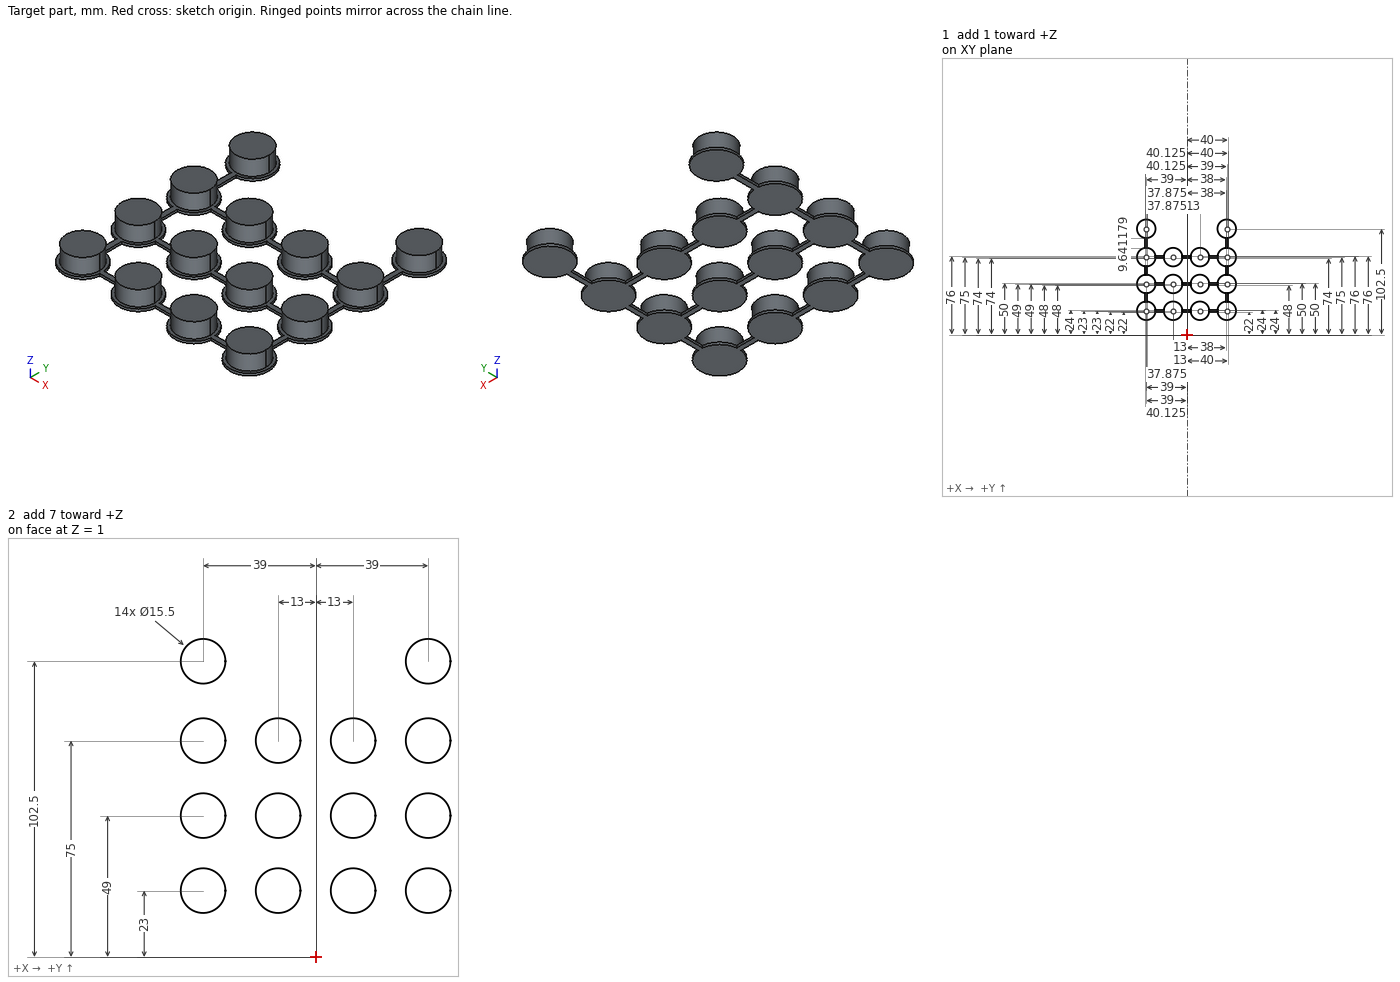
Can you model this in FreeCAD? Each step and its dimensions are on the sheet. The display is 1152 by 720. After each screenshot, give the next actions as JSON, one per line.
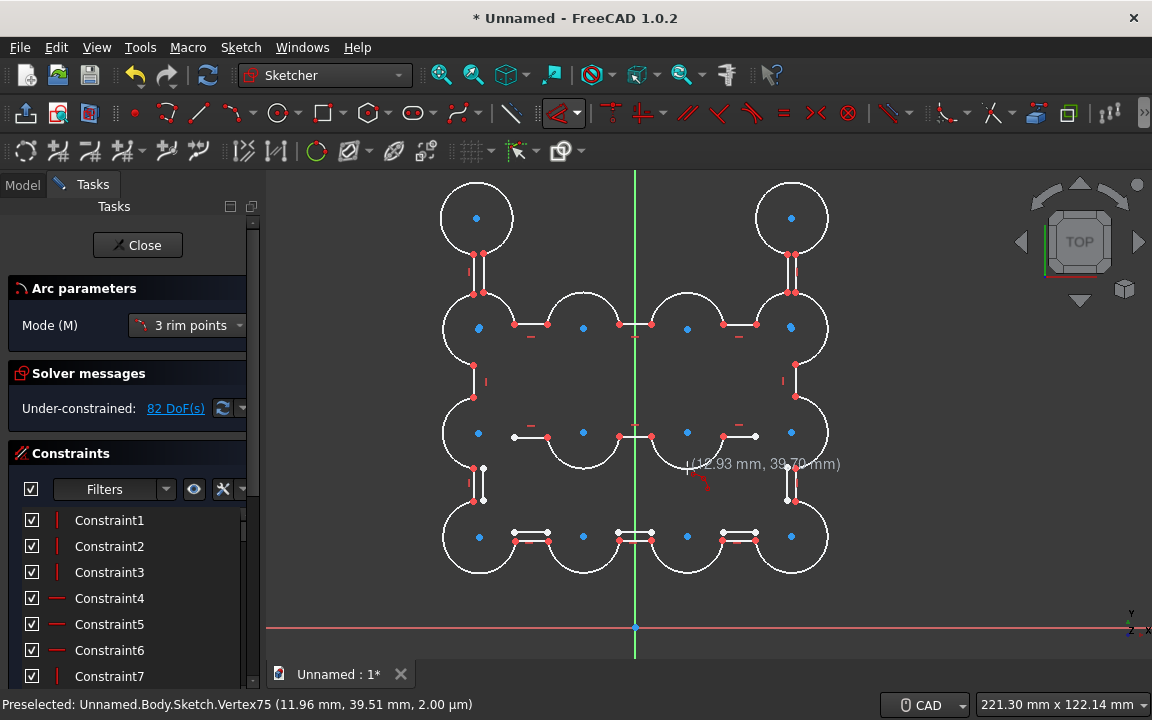
{"action": "left_click", "coordinate": [755, 437]}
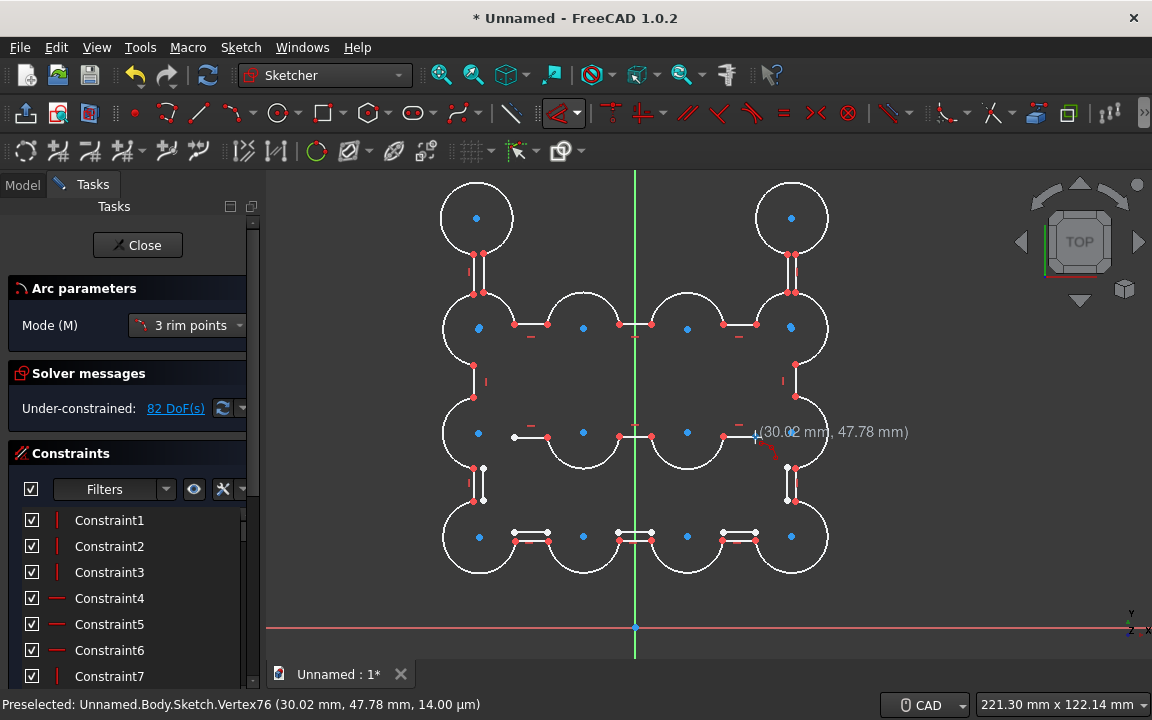
{"action": "scroll", "coordinate": [787, 468], "scroll_direction": "up", "scroll_amount": 4}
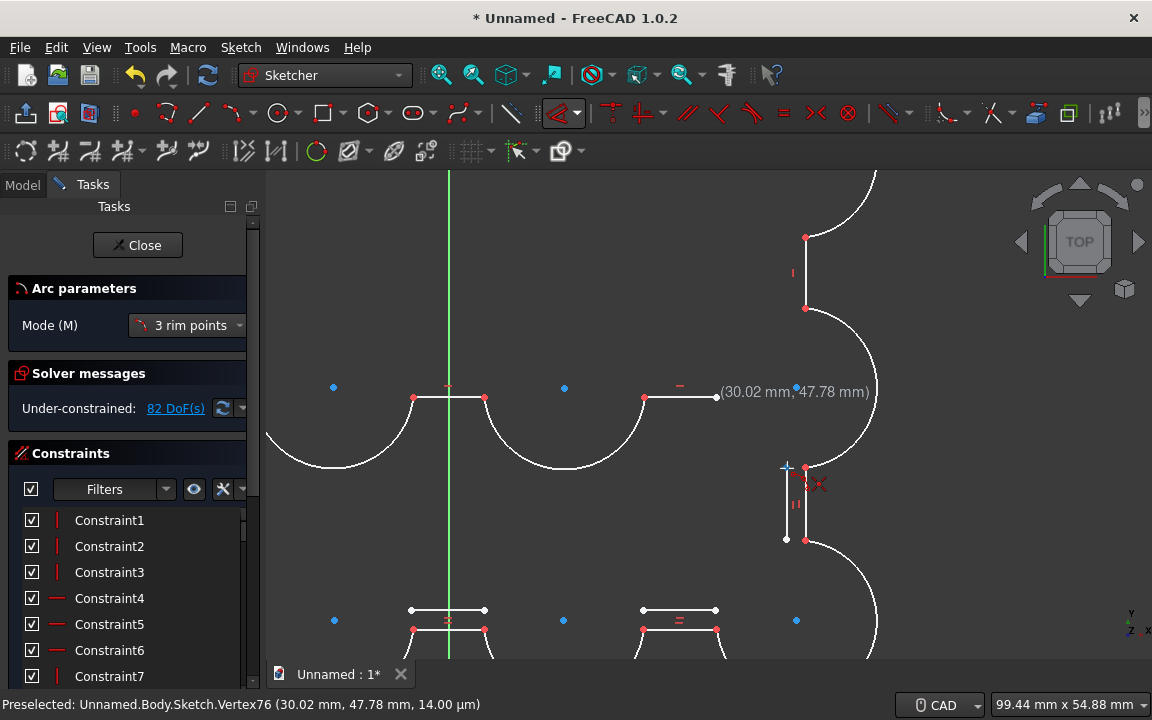
{"action": "left_click", "coordinate": [787, 467]}
{"action": "left_click", "coordinate": [739, 443]}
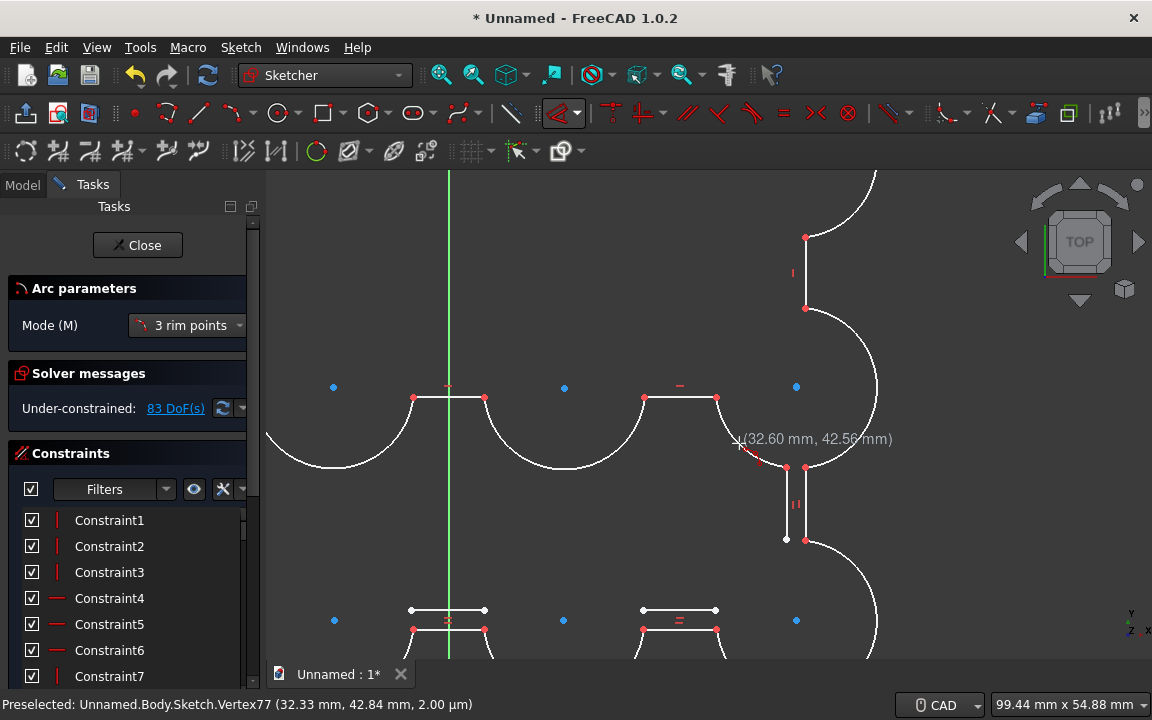
{"action": "left_click", "coordinate": [787, 539]}
{"action": "left_click", "coordinate": [716, 610]}
{"action": "left_click", "coordinate": [739, 562]}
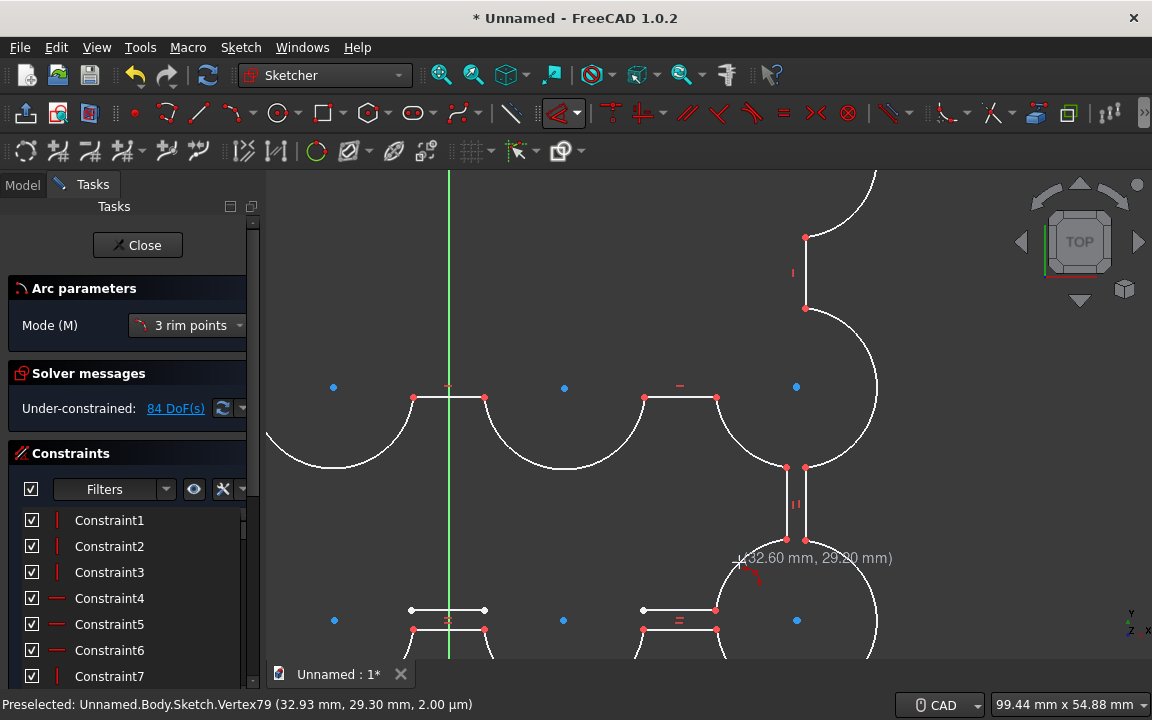
{"action": "left_click", "coordinate": [644, 610]}
{"action": "left_click", "coordinate": [485, 610]}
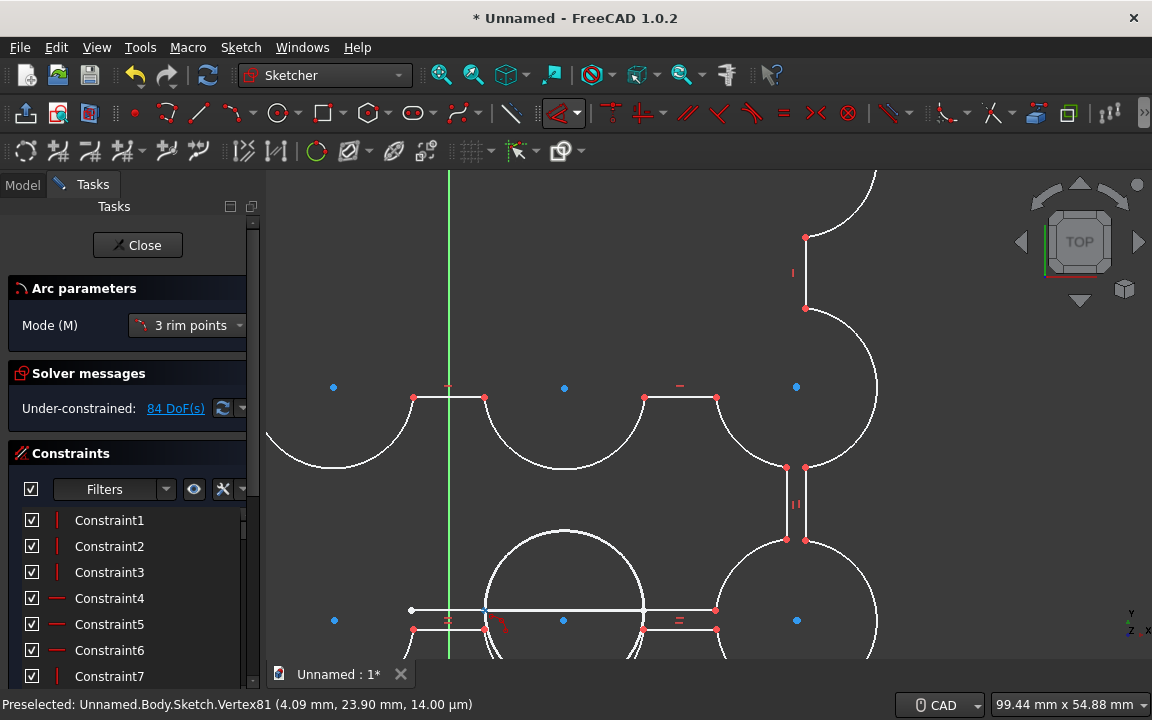
{"action": "scroll", "coordinate": [723, 452], "scroll_direction": "down", "scroll_amount": 6}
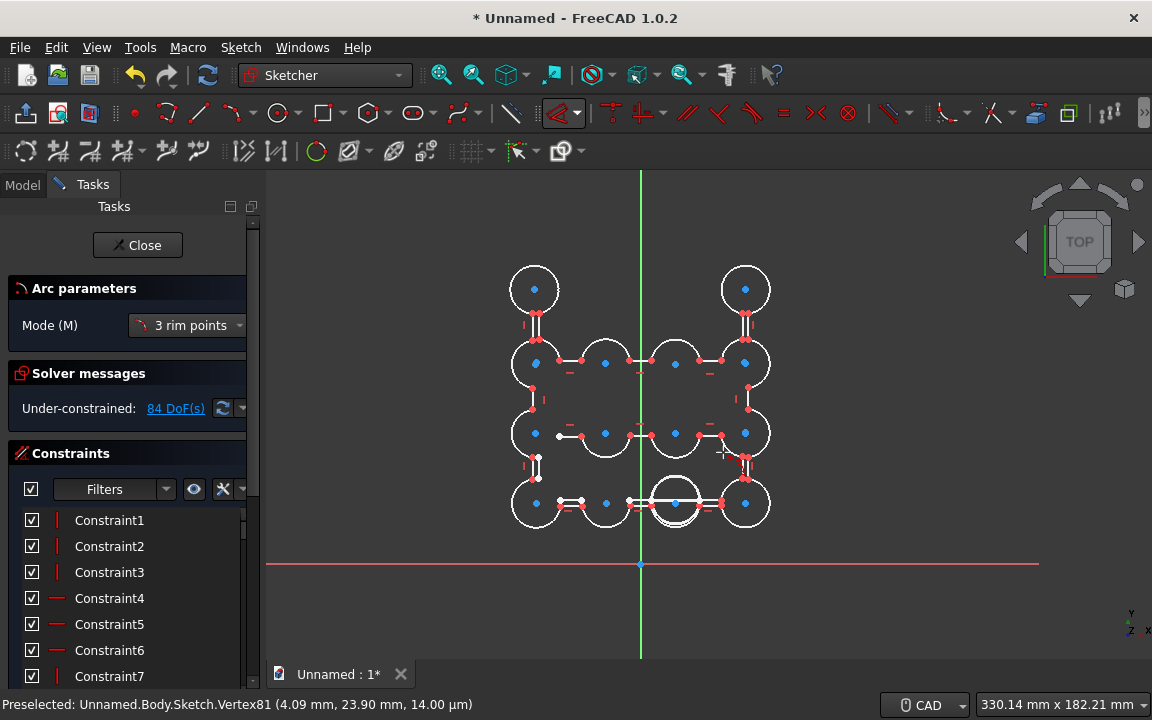
{"action": "left_click", "coordinate": [676, 478]}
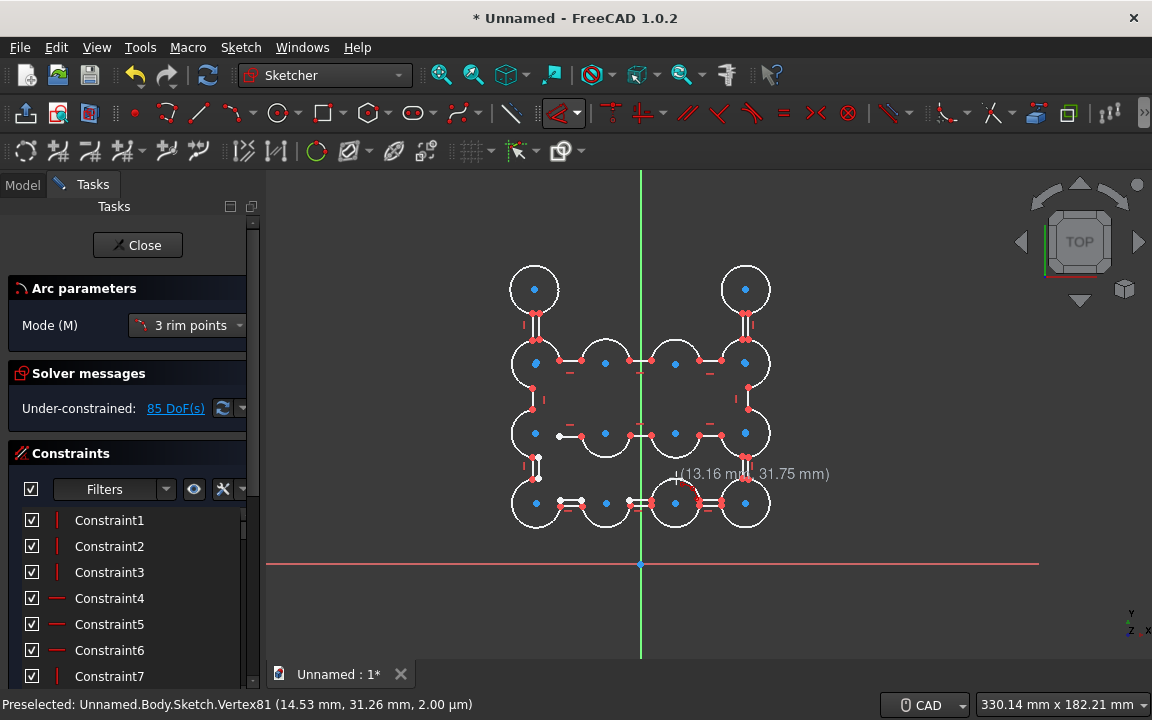
{"action": "scroll", "coordinate": [630, 500], "scroll_direction": "up", "scroll_amount": 6}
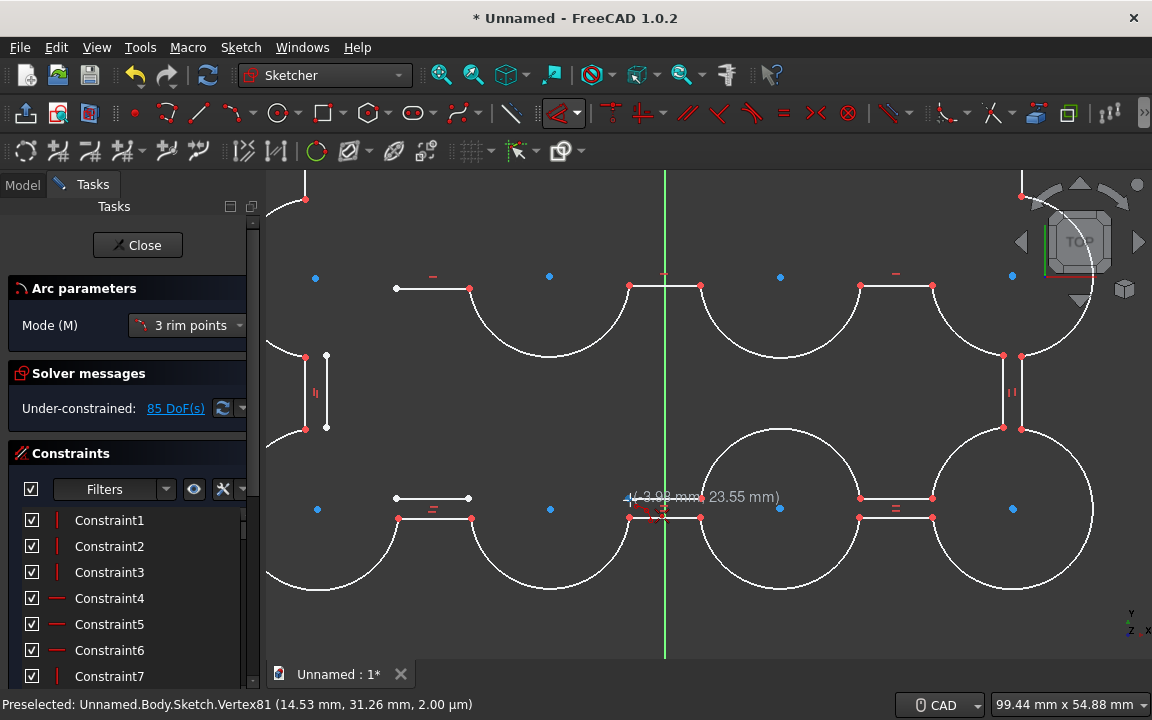
{"action": "left_click", "coordinate": [628, 499]}
{"action": "left_click", "coordinate": [469, 499]}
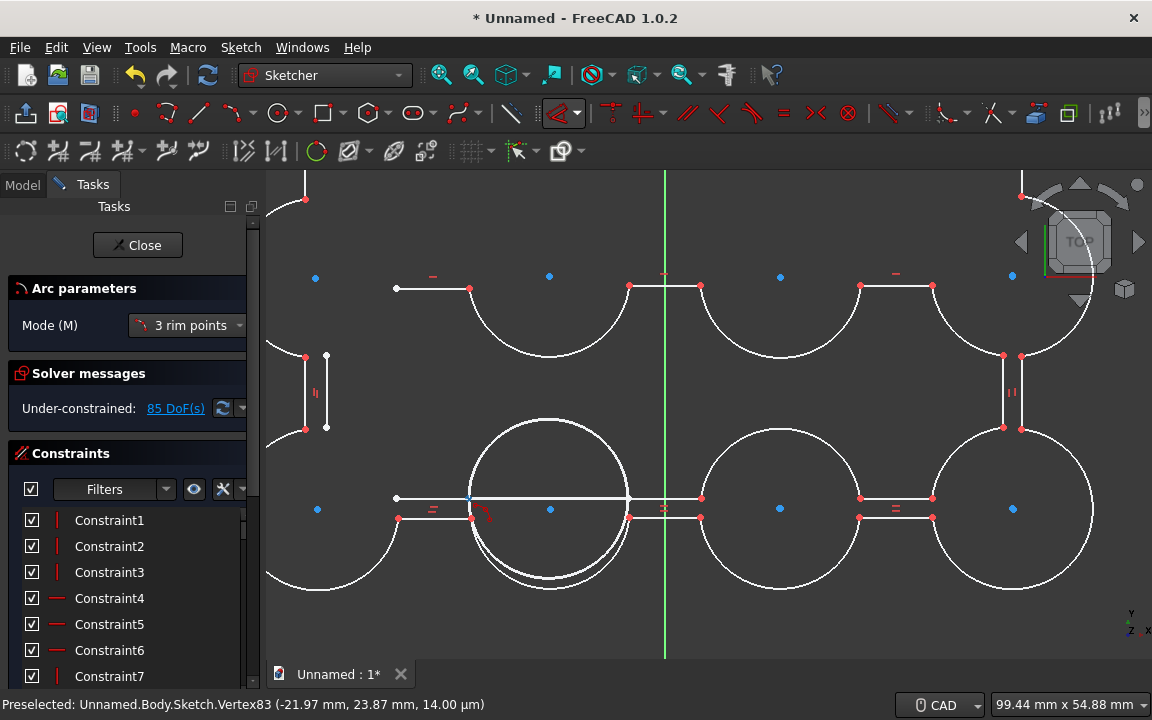
{"action": "scroll", "coordinate": [630, 501], "scroll_direction": "down", "scroll_amount": 6}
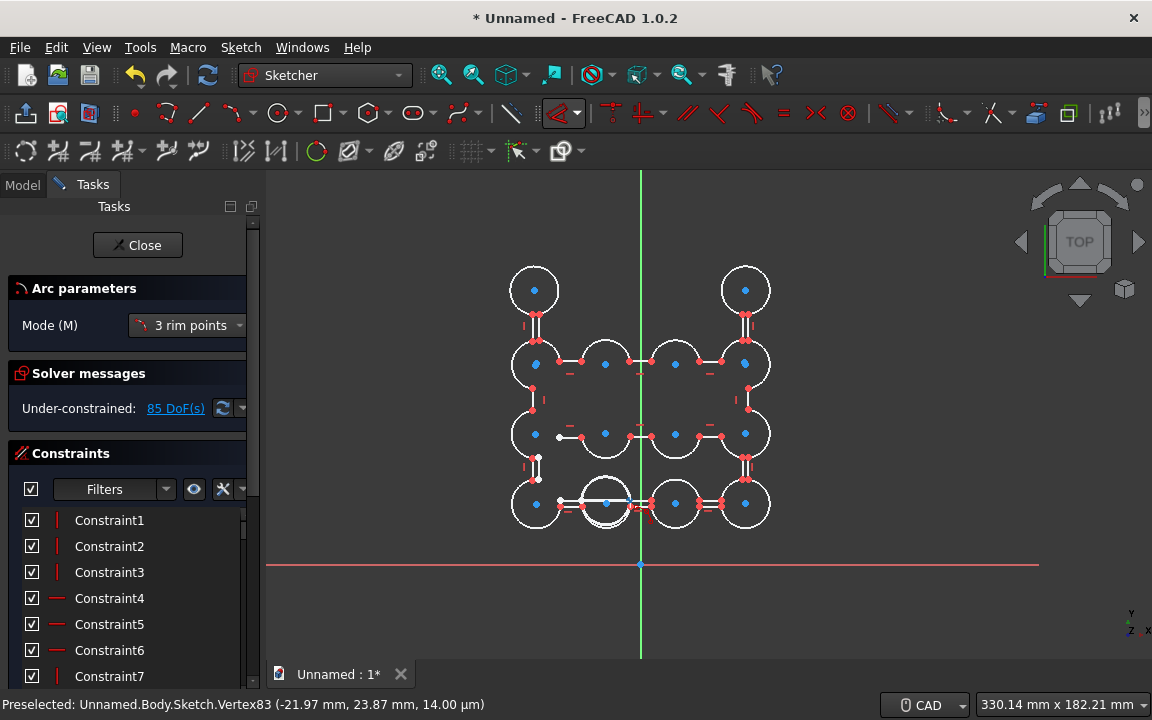
{"action": "left_click", "coordinate": [606, 479]}